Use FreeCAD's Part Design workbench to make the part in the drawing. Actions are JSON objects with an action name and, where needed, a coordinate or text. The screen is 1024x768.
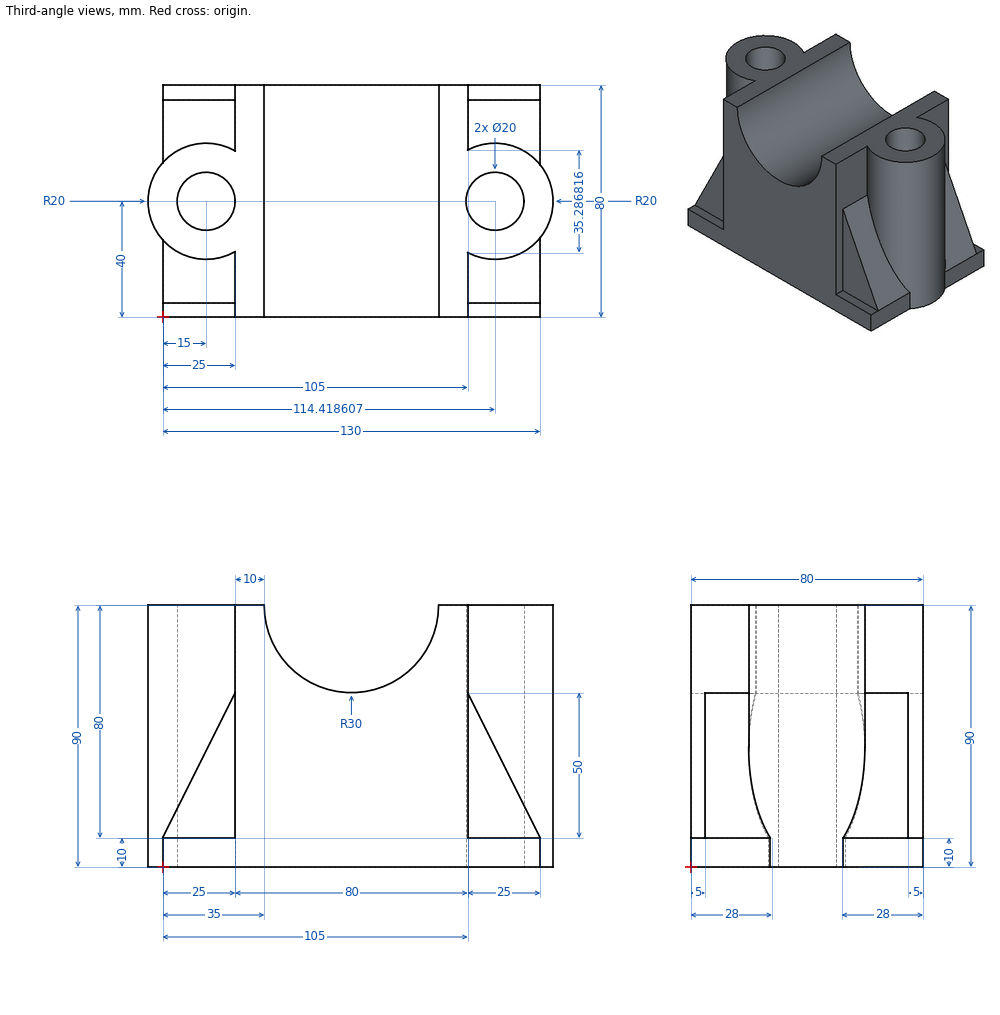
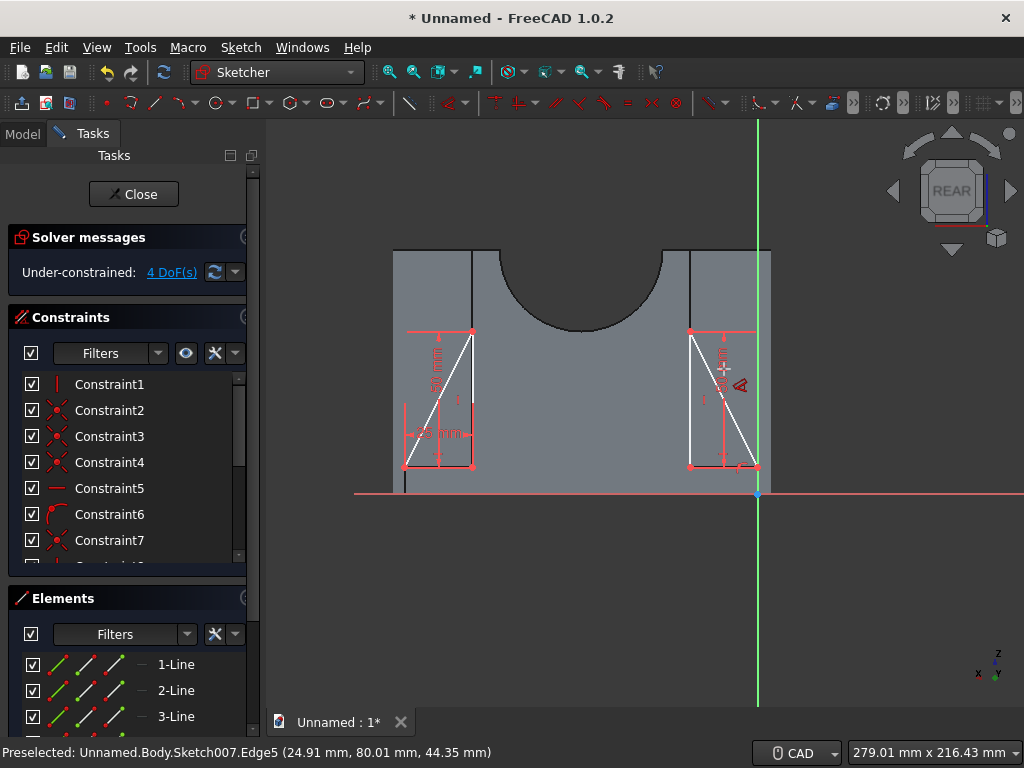
{"action": "left_click", "coordinate": [710, 468]}
{"action": "left_click", "coordinate": [724, 434]}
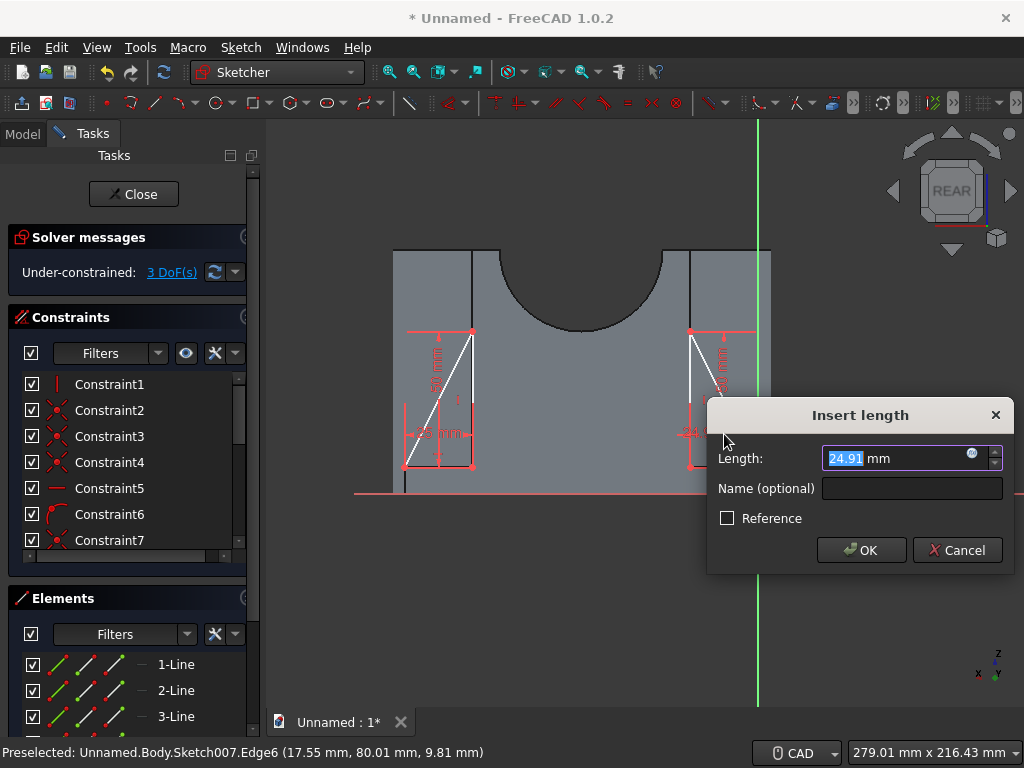
{"action": "type", "text": "25"}
{"action": "key", "text": "Return"}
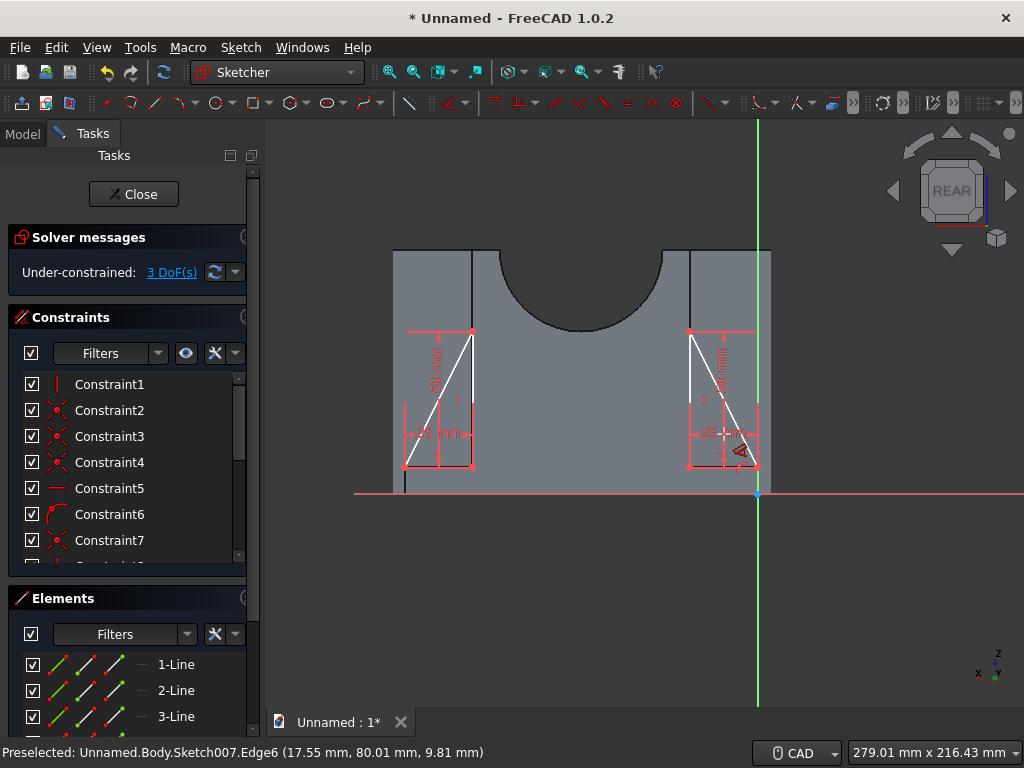
{"action": "scroll", "coordinate": [473, 468], "scroll_direction": "up", "scroll_amount": 2}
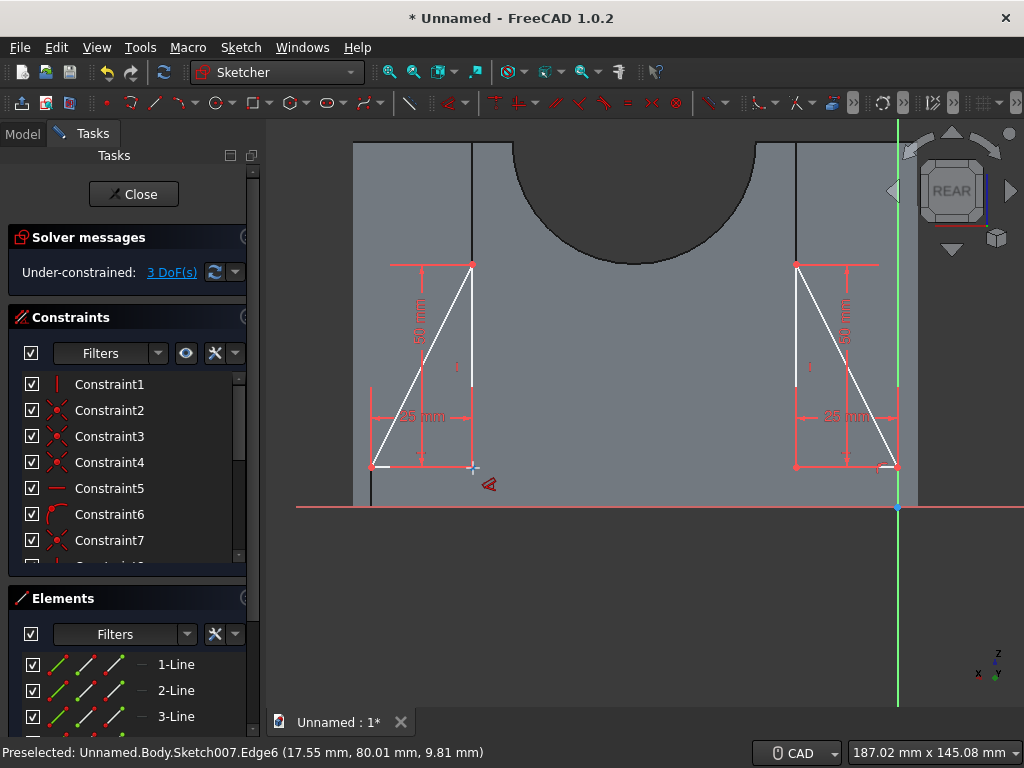
{"action": "left_click", "coordinate": [472, 467]}
{"action": "left_click", "coordinate": [438, 487]}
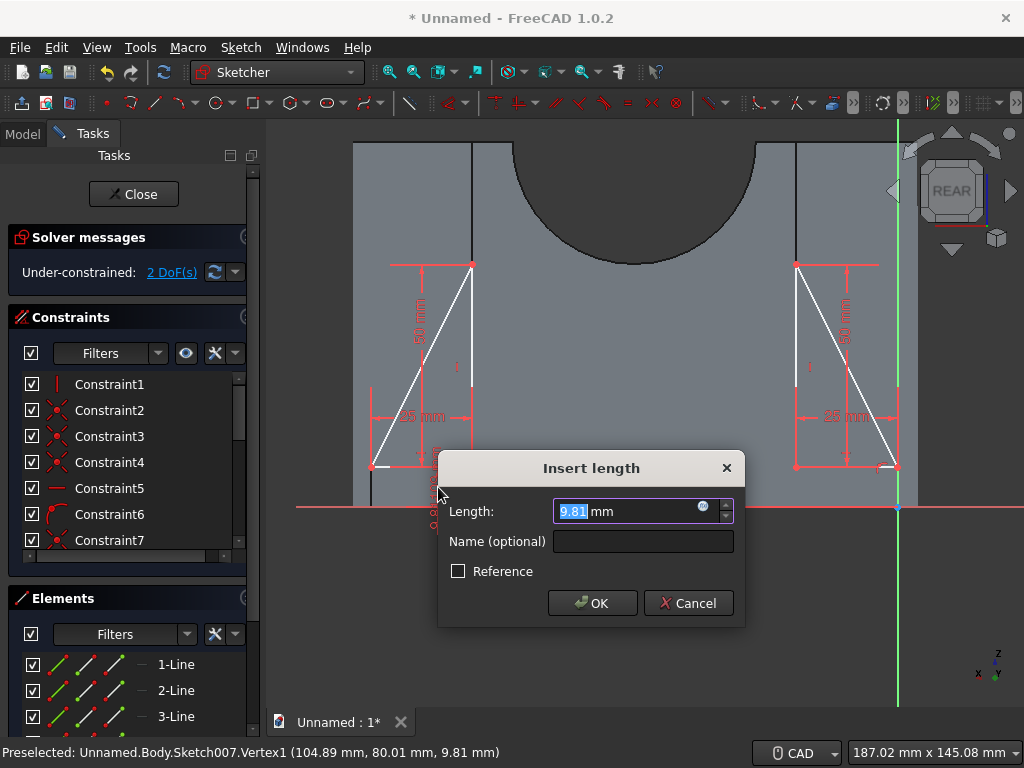
{"action": "type", "text": "10"}
{"action": "key", "text": "Return"}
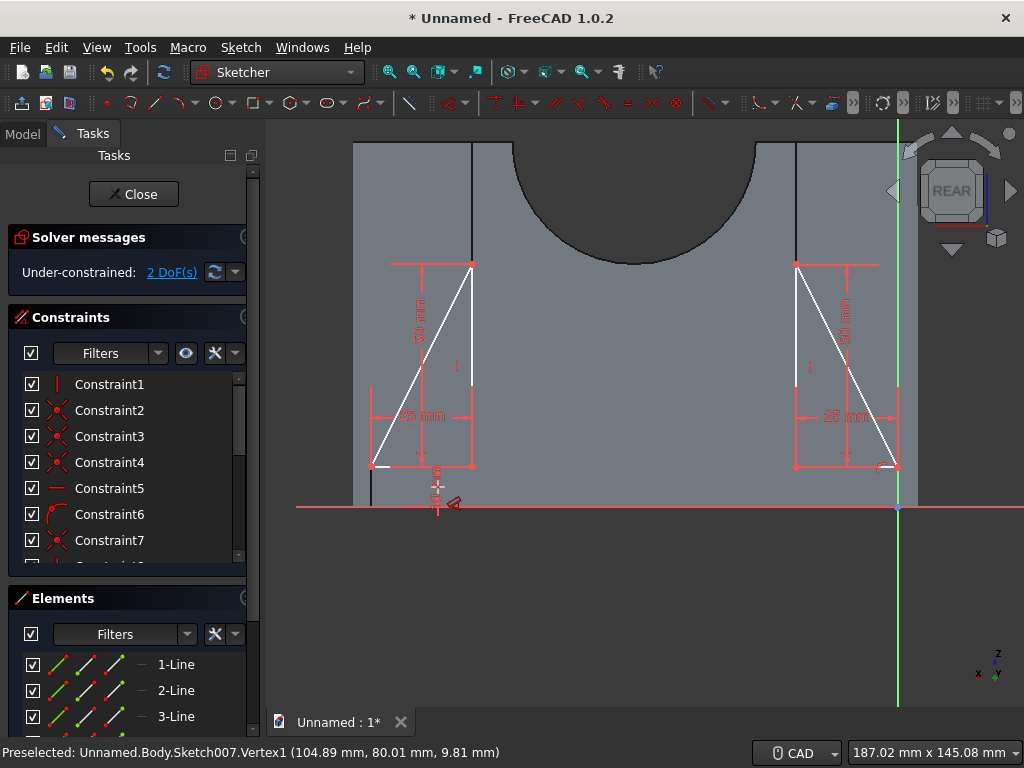
{"action": "scroll", "coordinate": [316, 537], "scroll_direction": "down", "scroll_amount": 1}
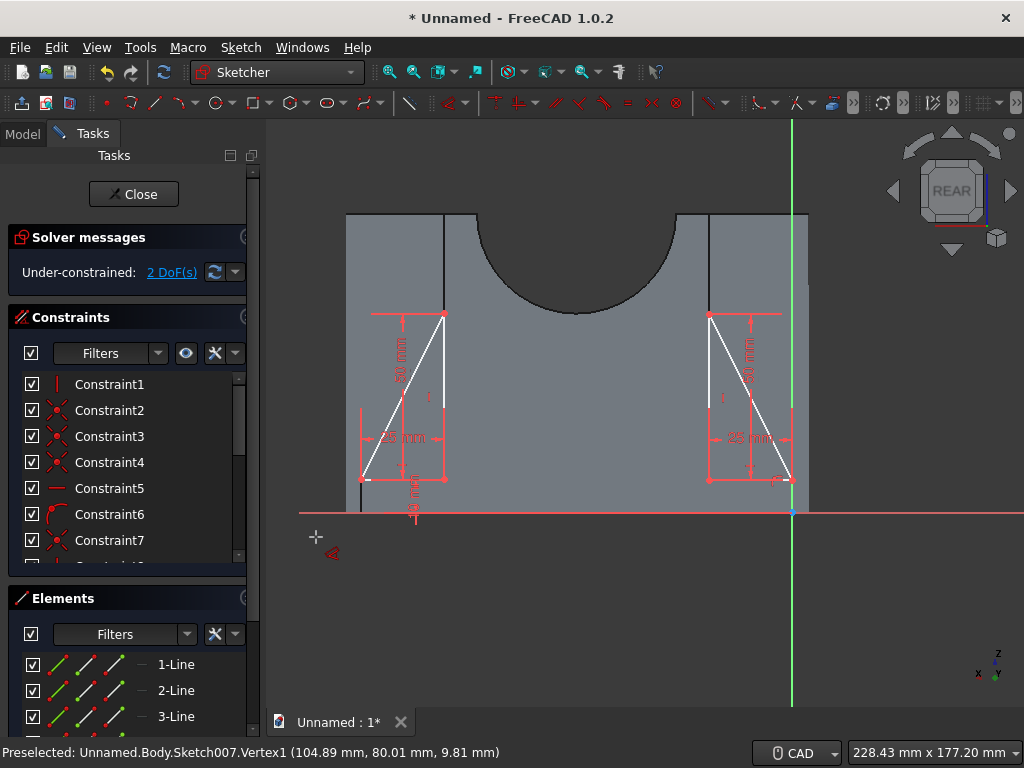
{"action": "left_click", "coordinate": [792, 480]}
{"action": "left_click", "coordinate": [826, 496]}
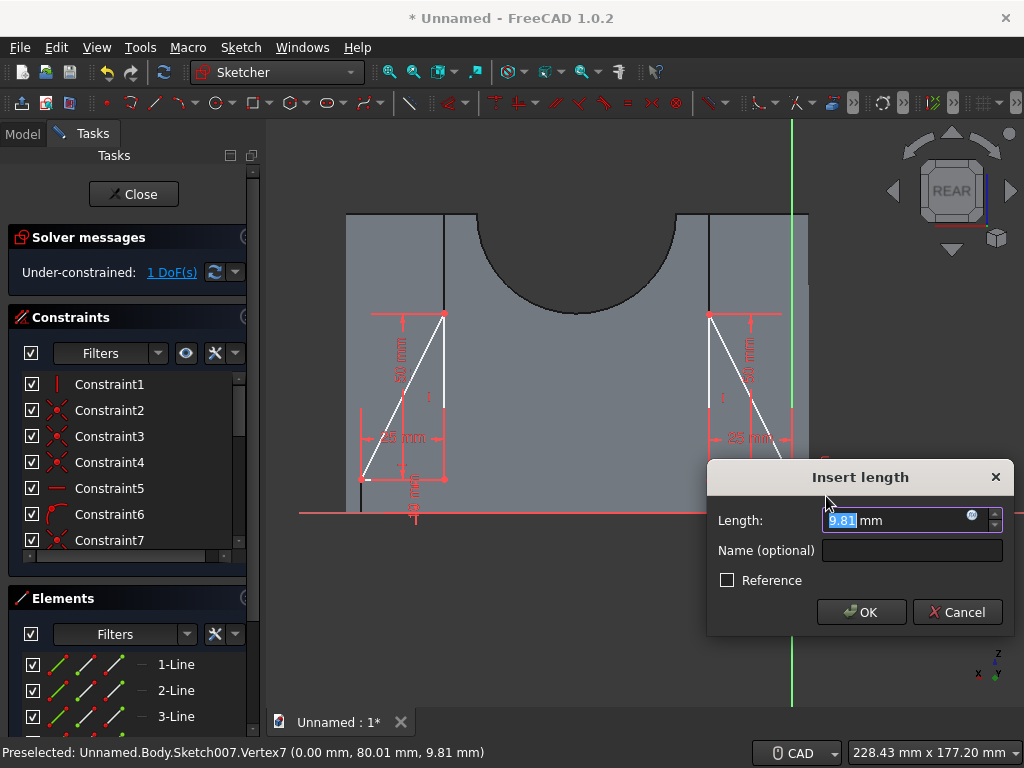
{"action": "type", "text": "10"}
{"action": "key", "text": "Return"}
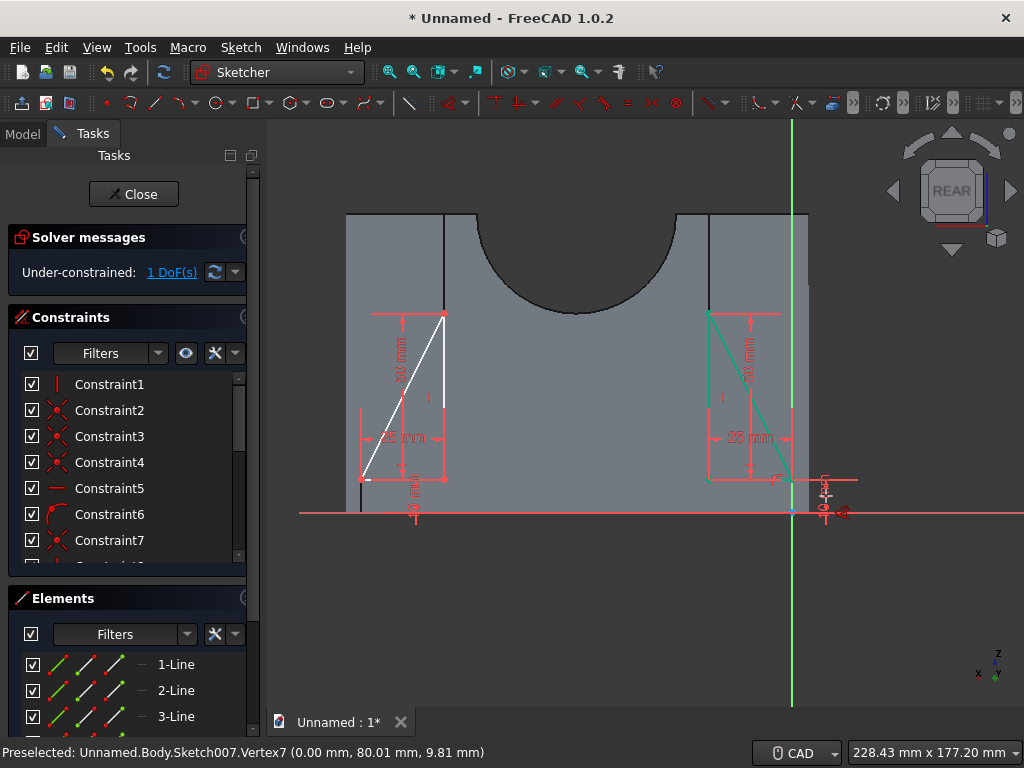
{"action": "left_click", "coordinate": [444, 480]}
{"action": "left_click", "coordinate": [618, 547]}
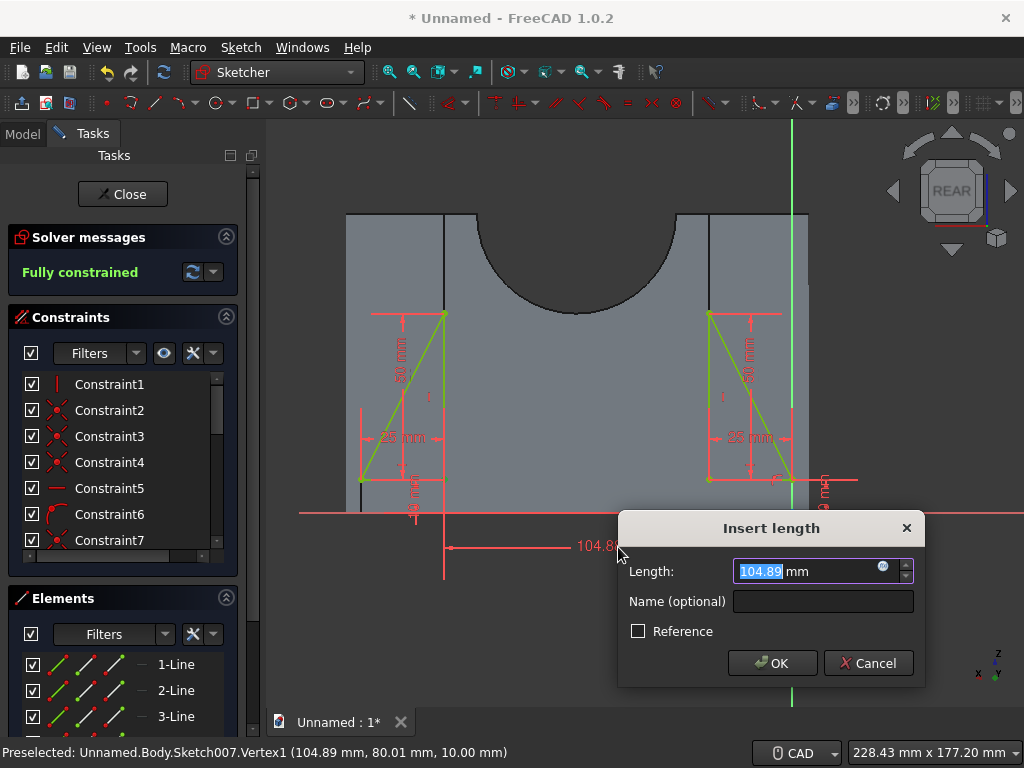
{"action": "type", "text": "105"}
{"action": "key", "text": "Return"}
{"action": "key", "text": "Escape"}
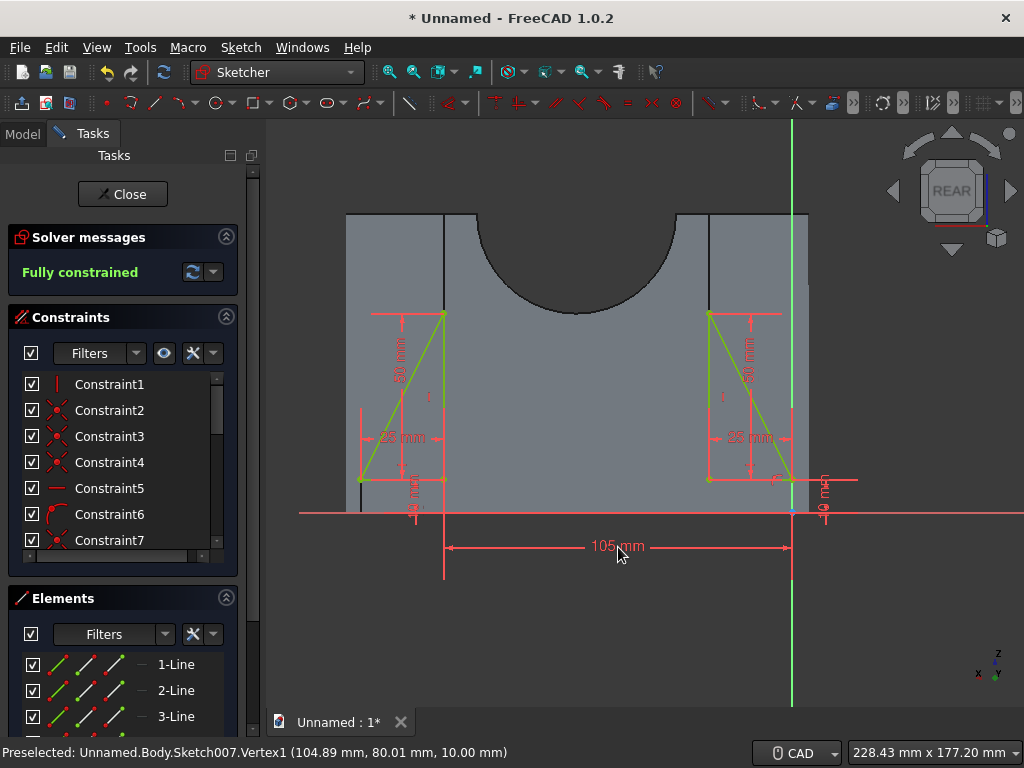
{"action": "left_click", "coordinate": [123, 194]}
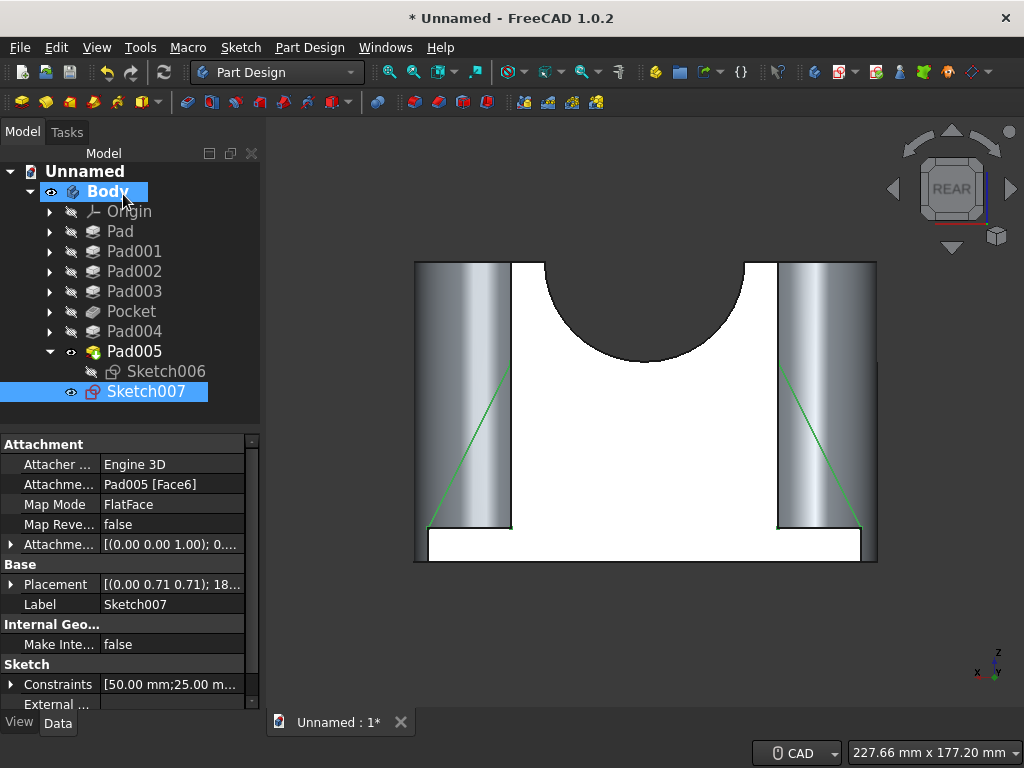
{"action": "left_click", "coordinate": [22, 102]}